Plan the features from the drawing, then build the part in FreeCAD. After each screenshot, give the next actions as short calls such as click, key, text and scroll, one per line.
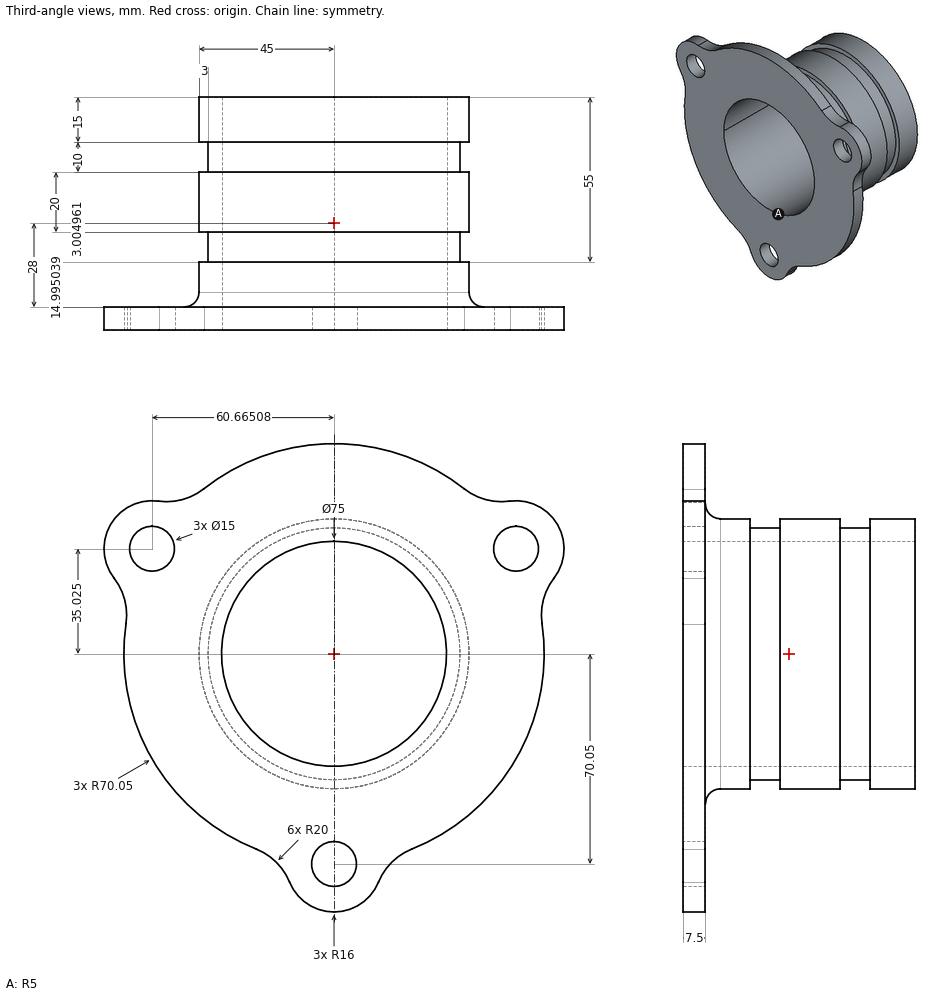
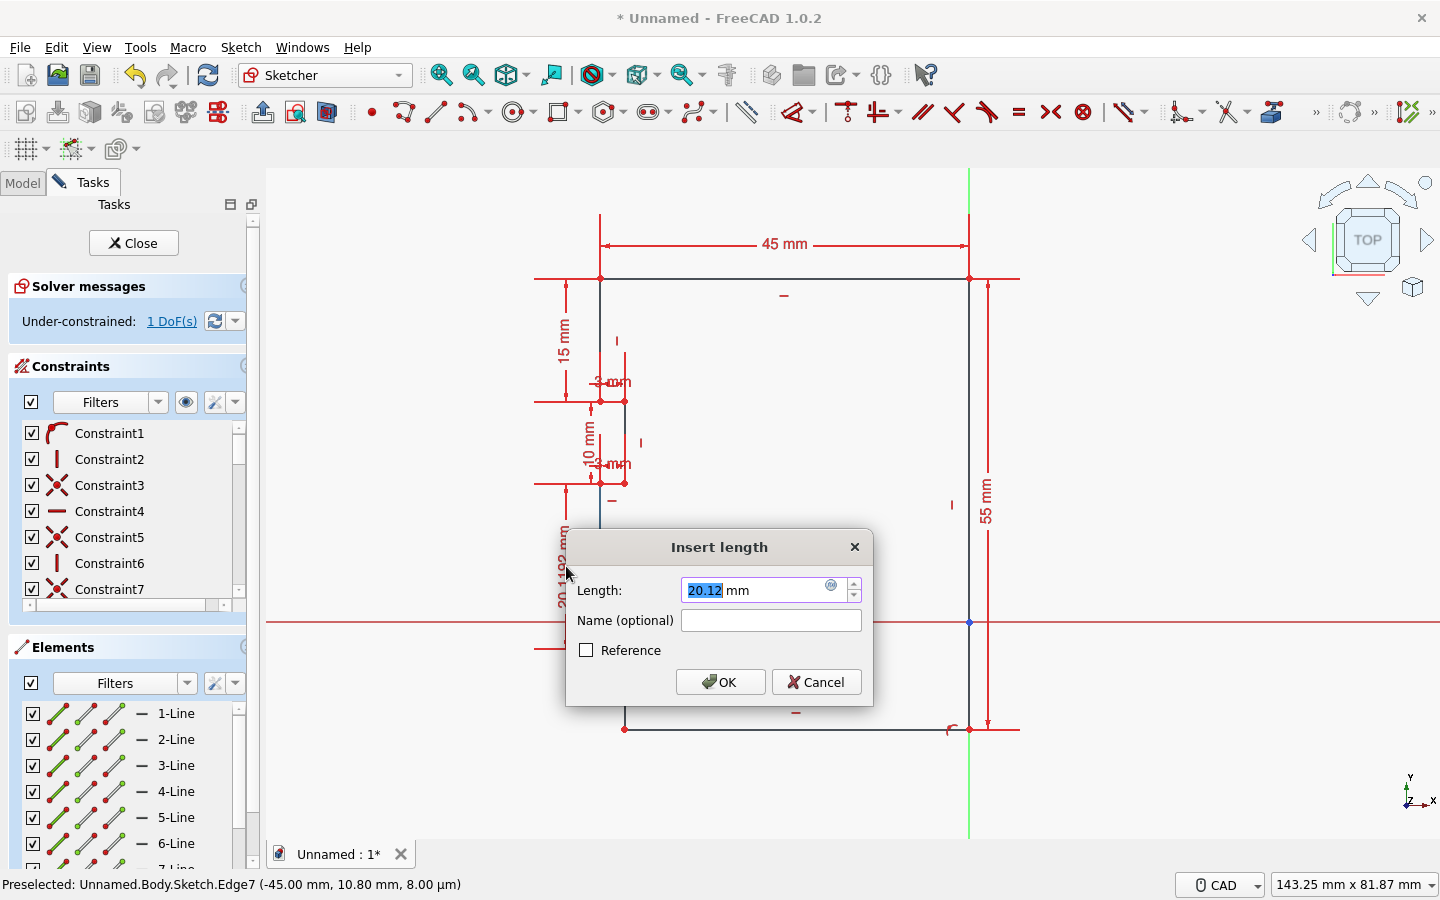
text(20)
key(Return)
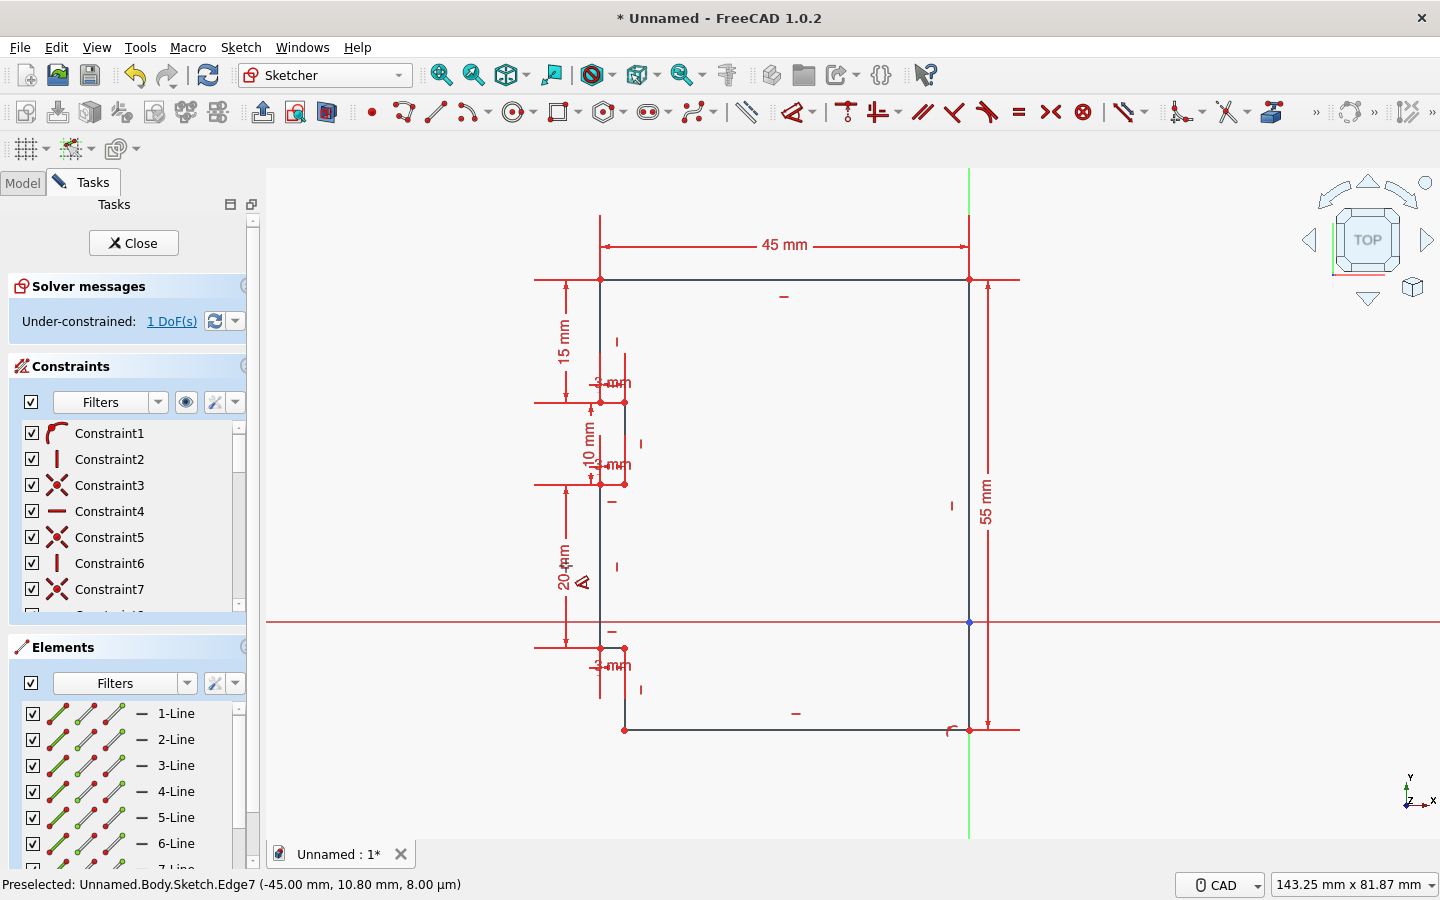
scroll(600, 648, up, 3)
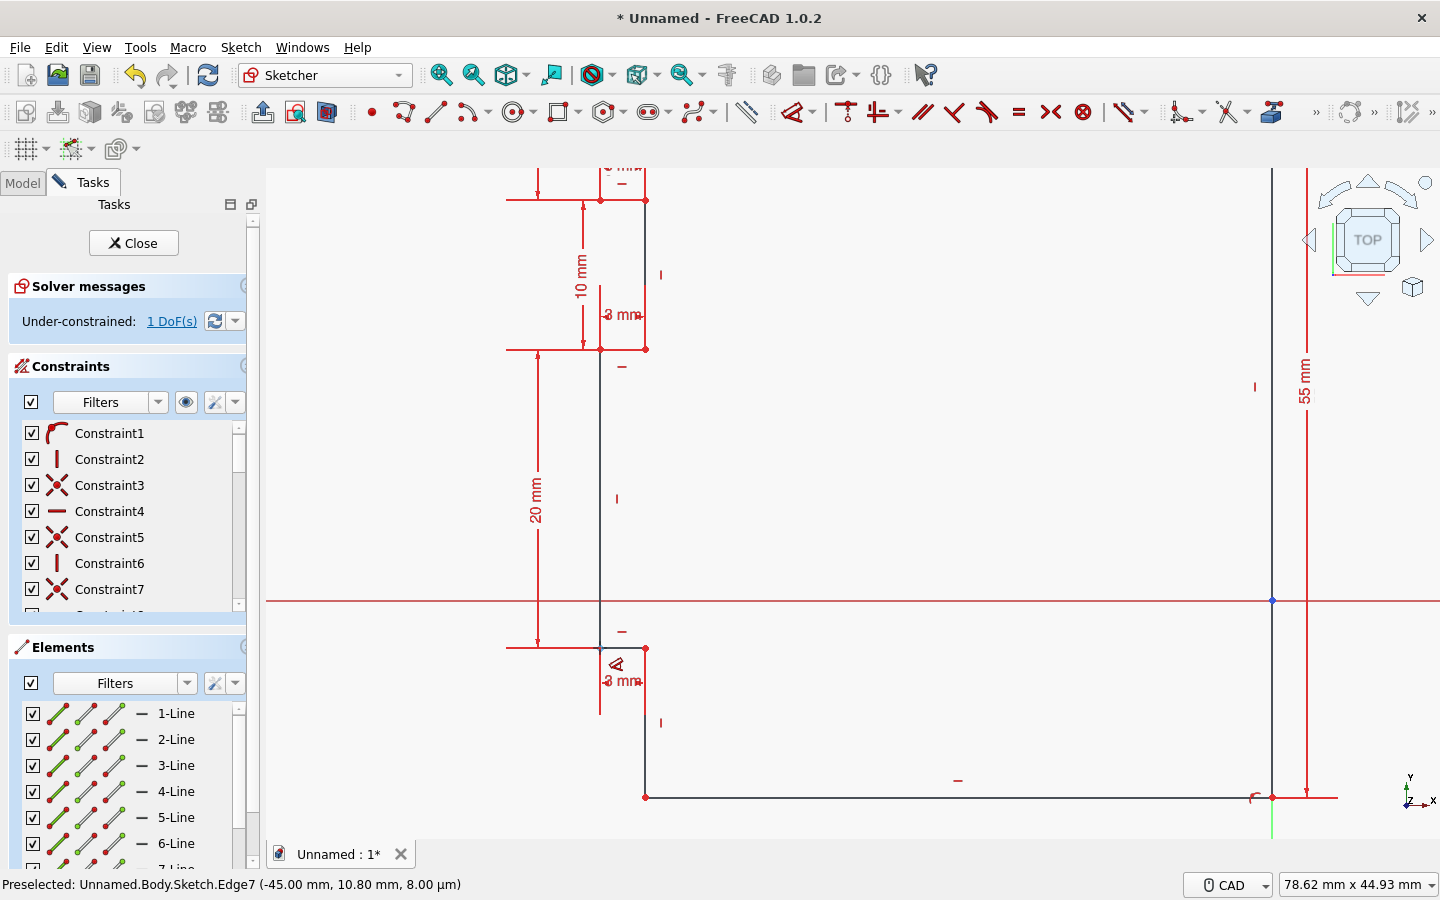
click(600, 648)
click(566, 625)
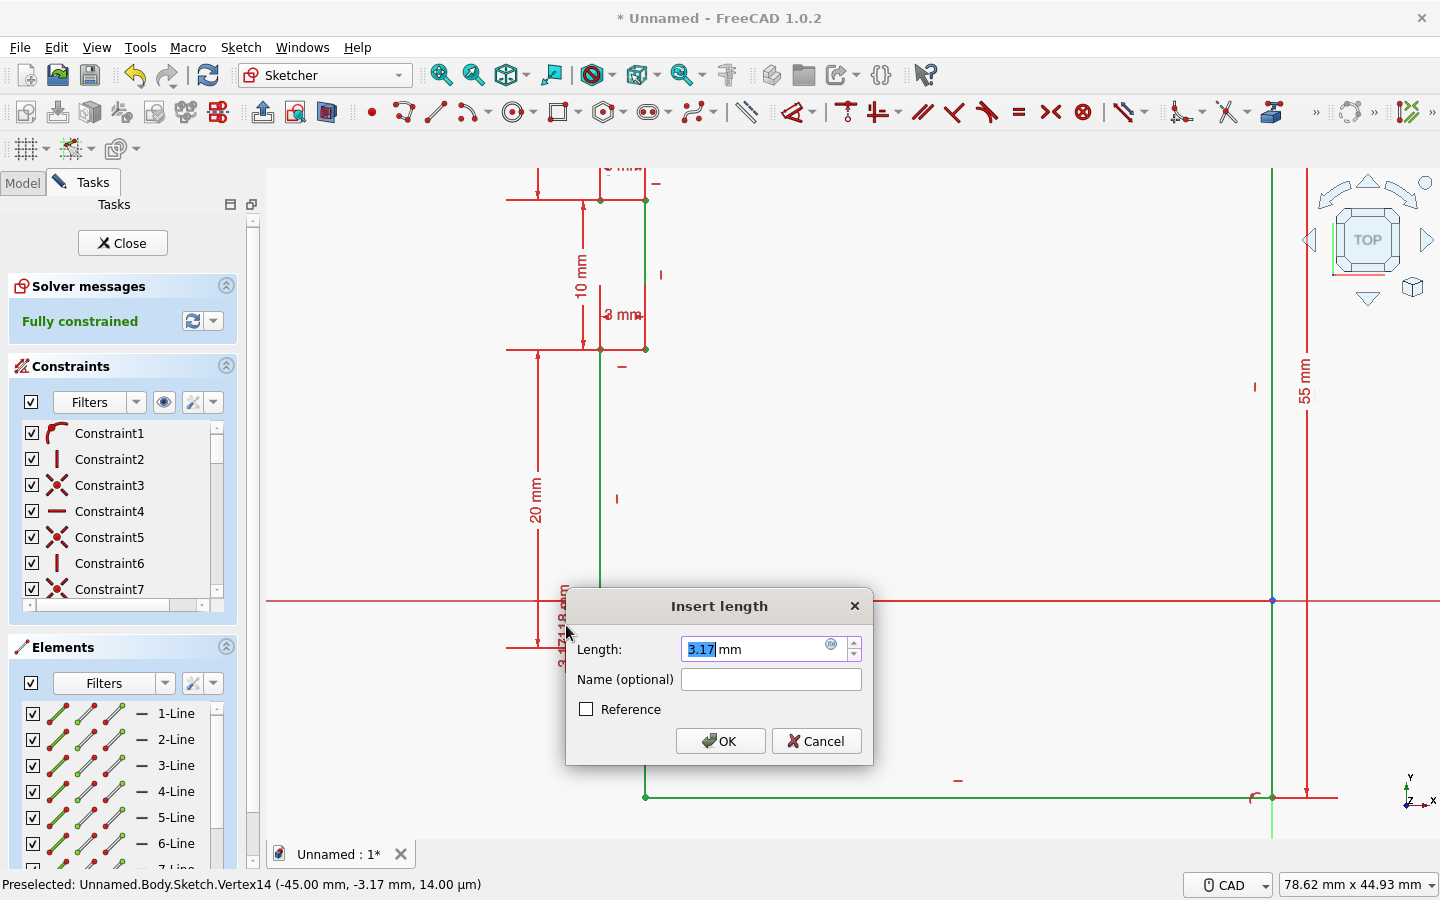
text(3.004961)
key(Return)
key(Escape)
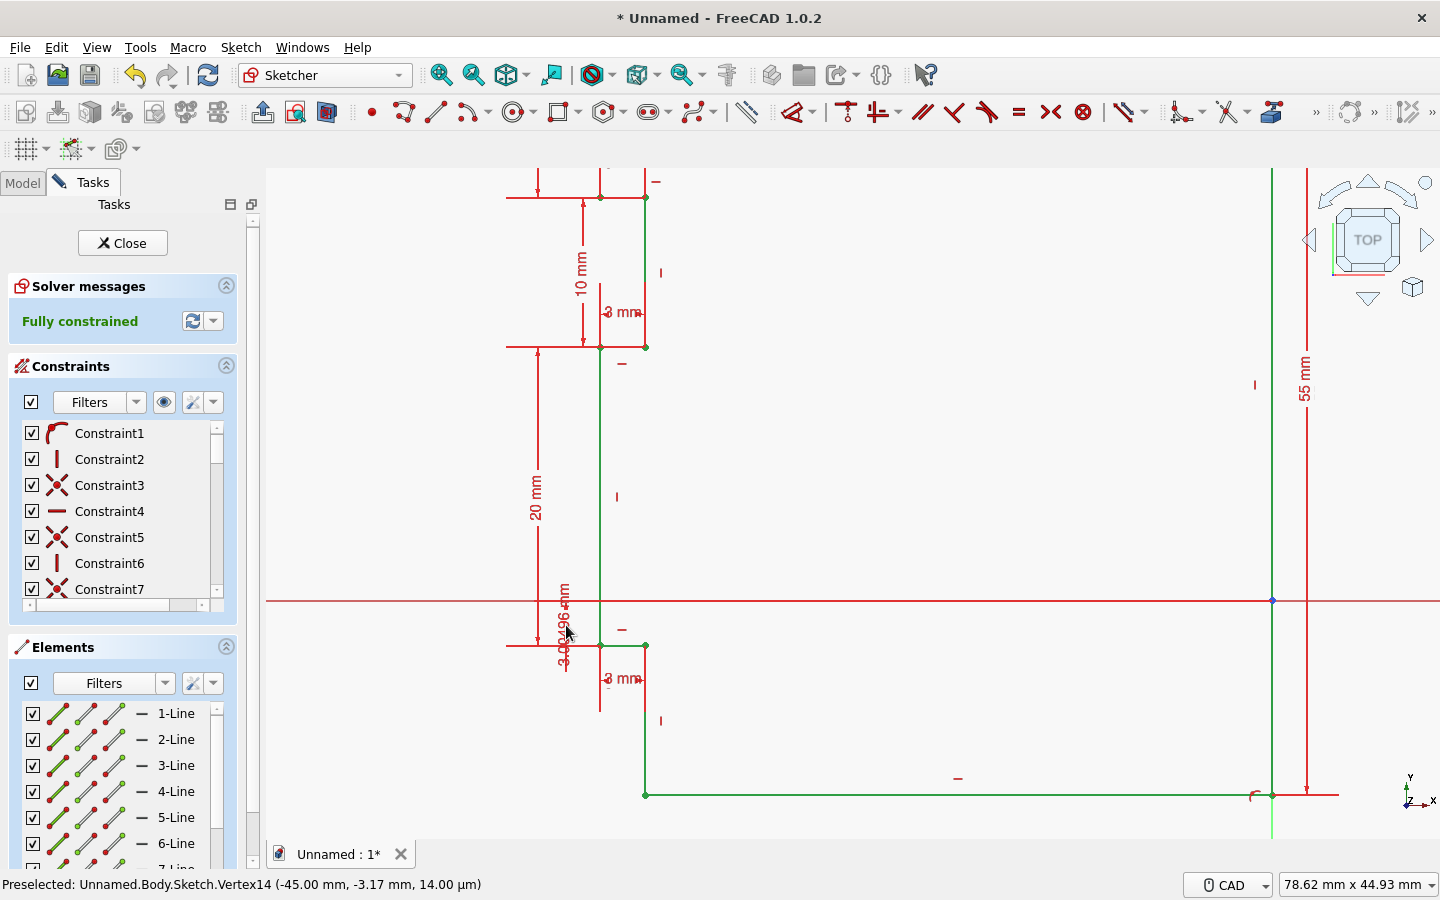
click(123, 243)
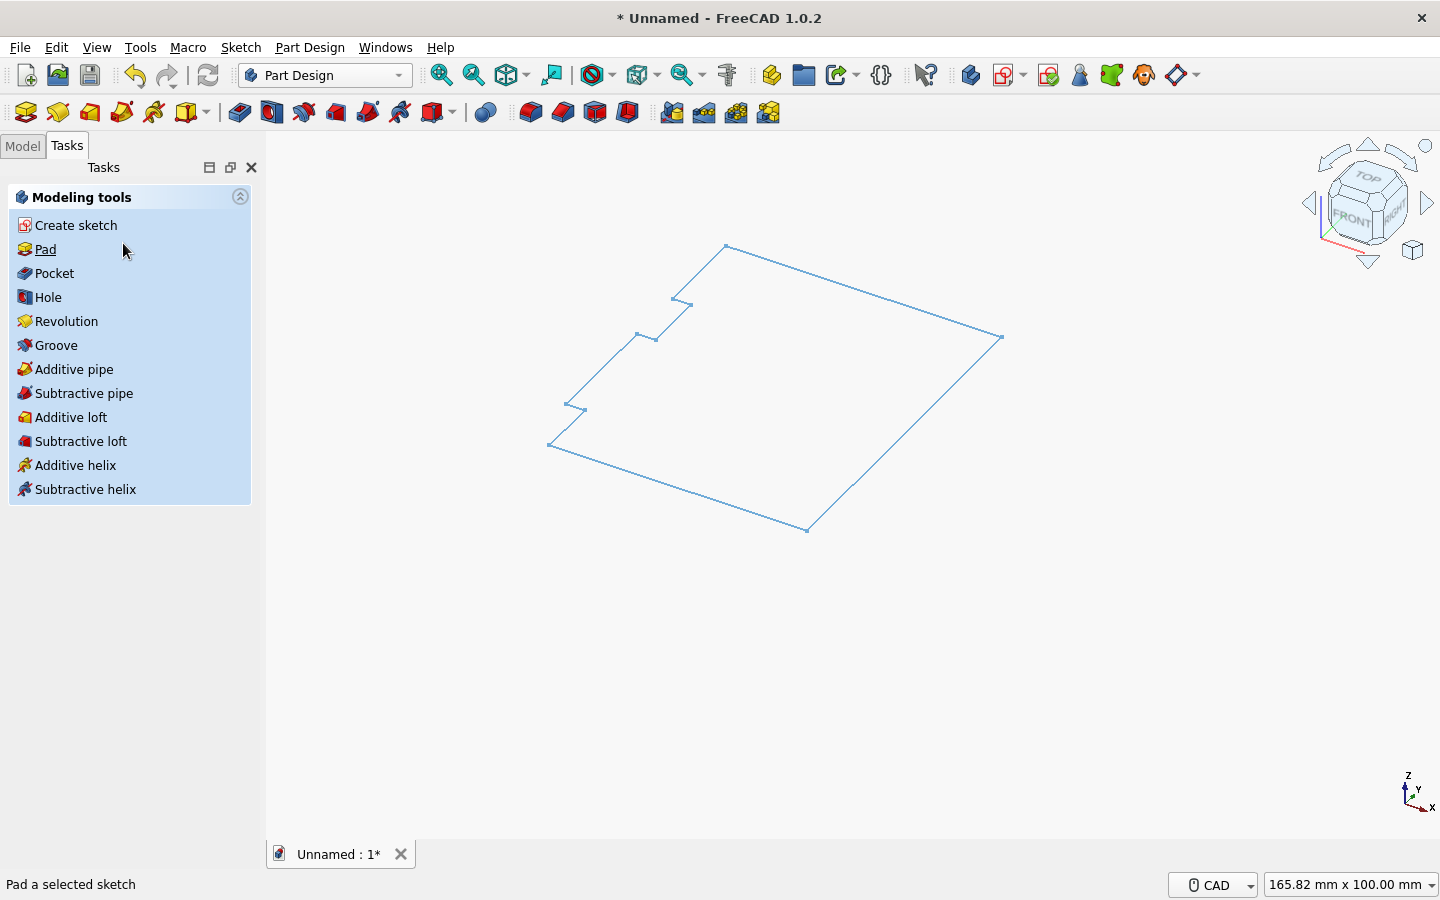
click(58, 112)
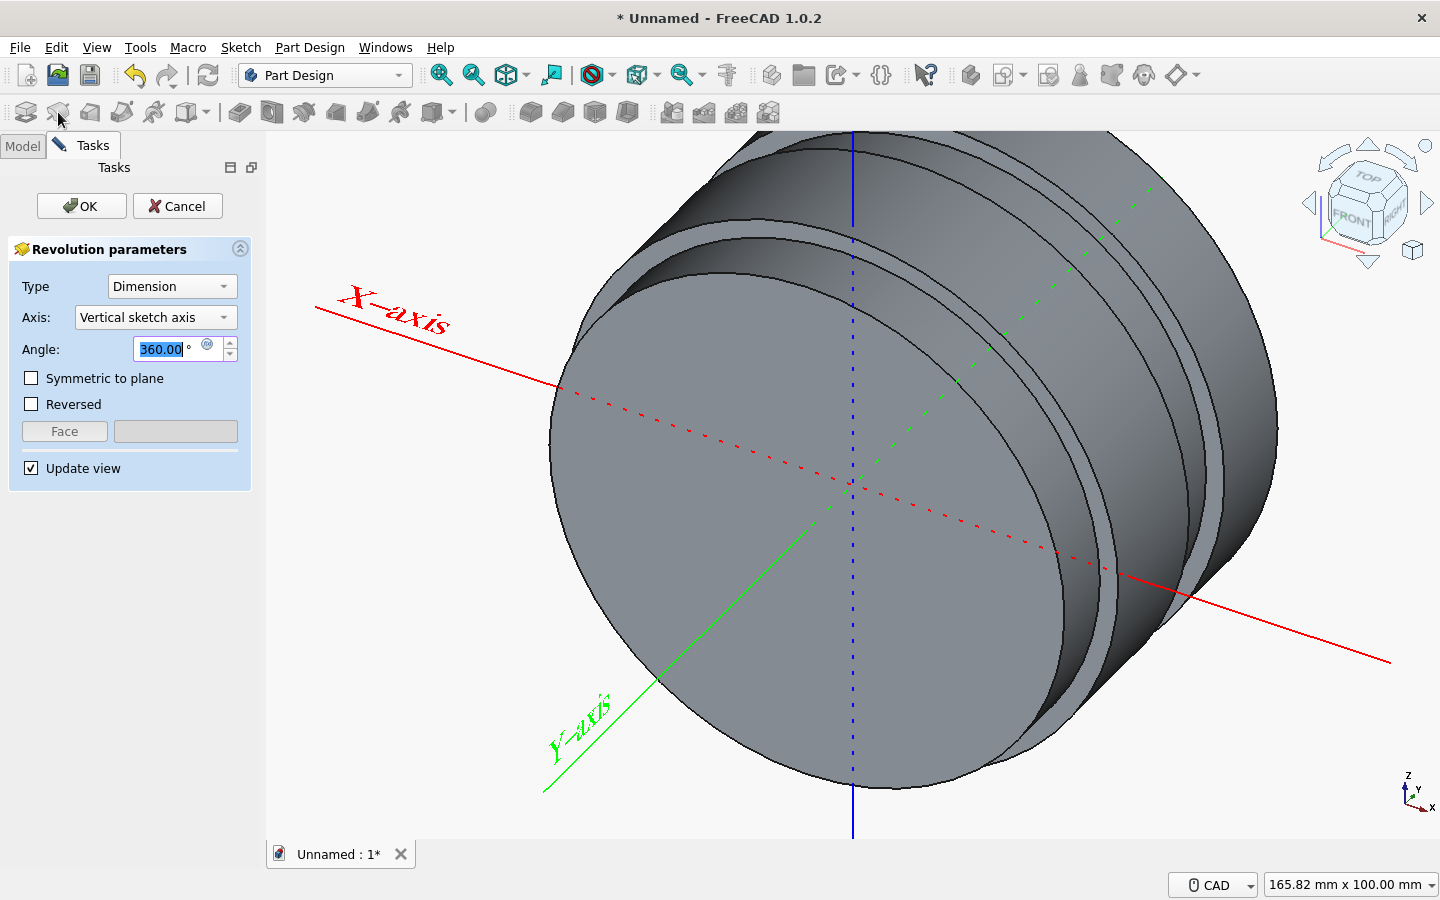
click(82, 206)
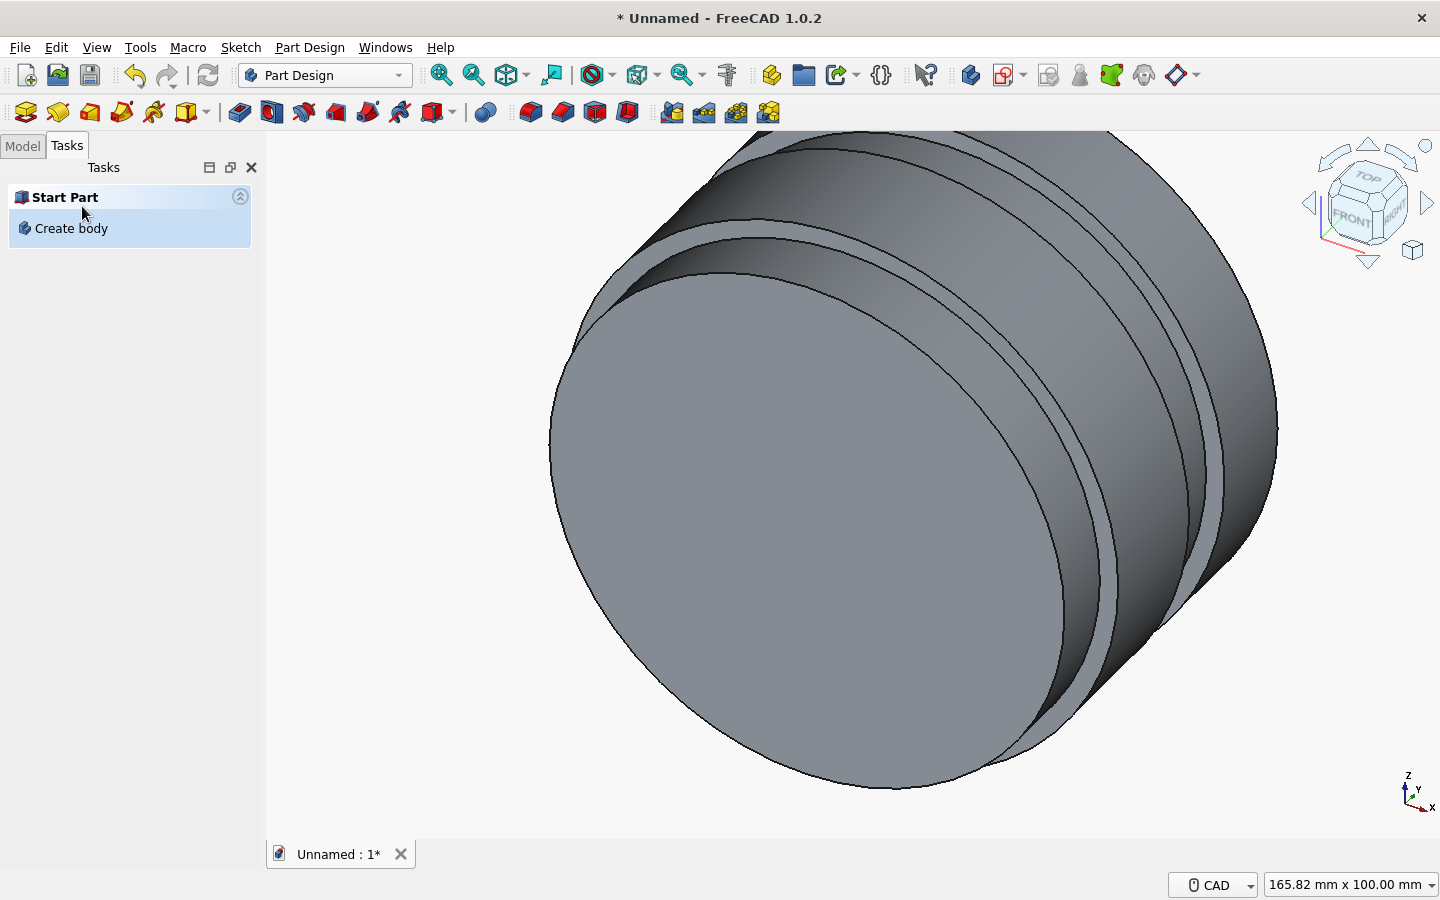
key(v)
key(f)